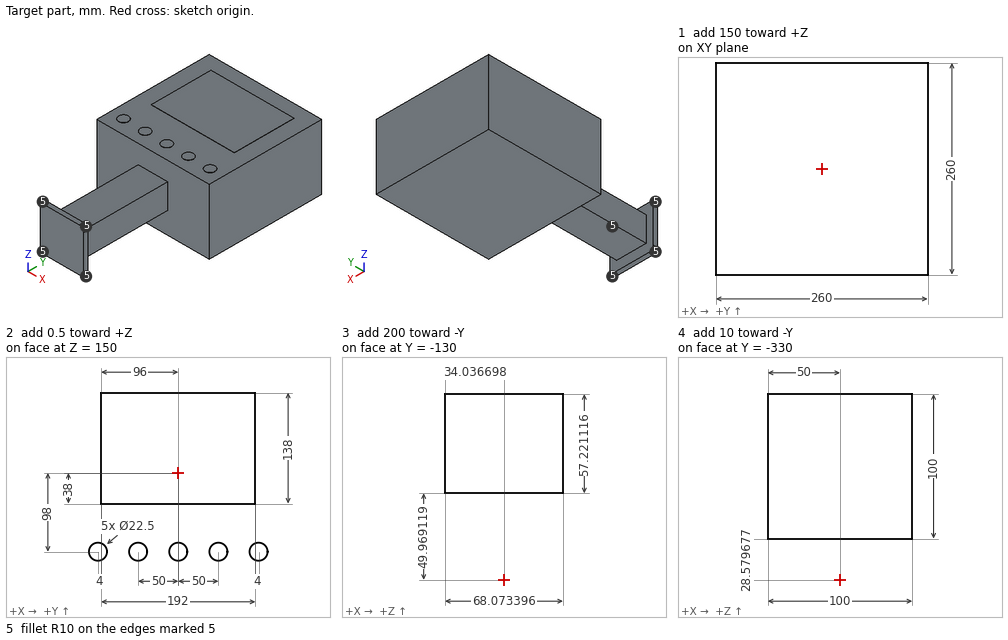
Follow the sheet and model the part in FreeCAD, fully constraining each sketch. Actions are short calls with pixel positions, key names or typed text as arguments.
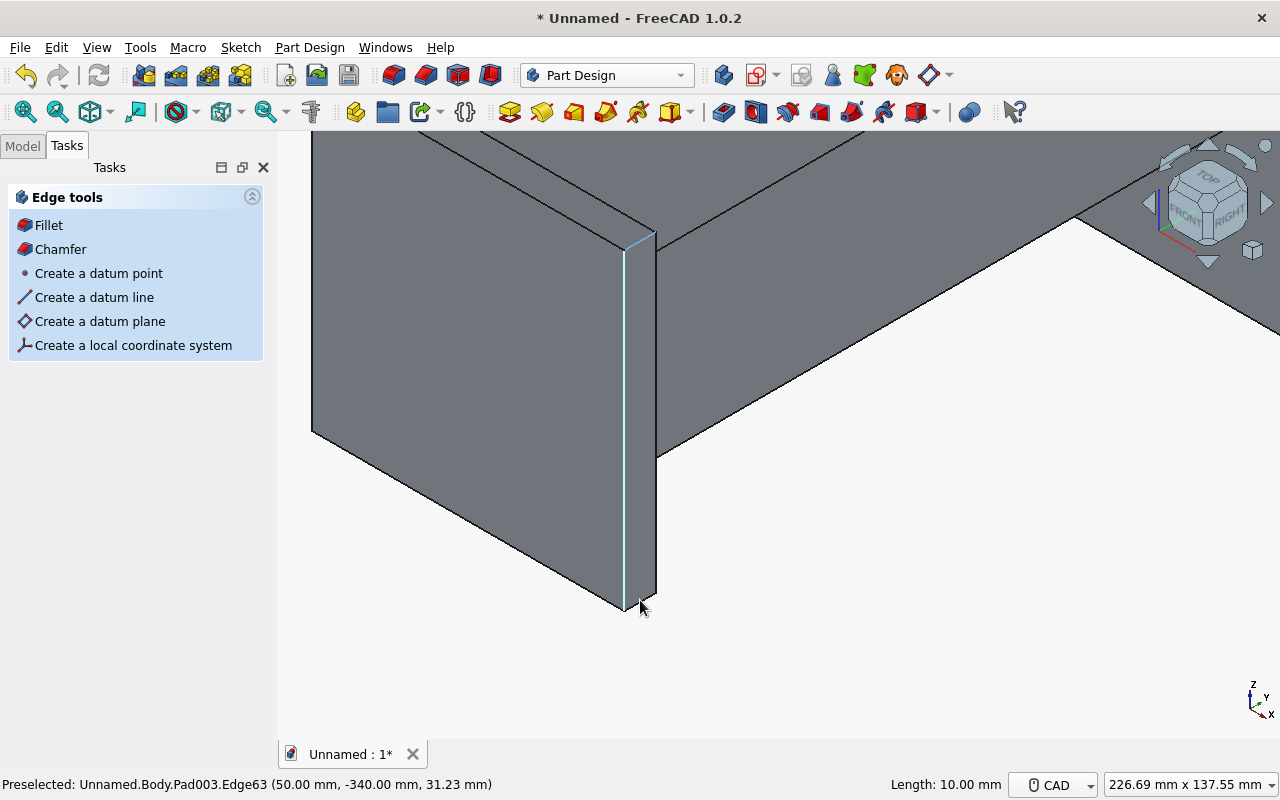
key(v)
key(f)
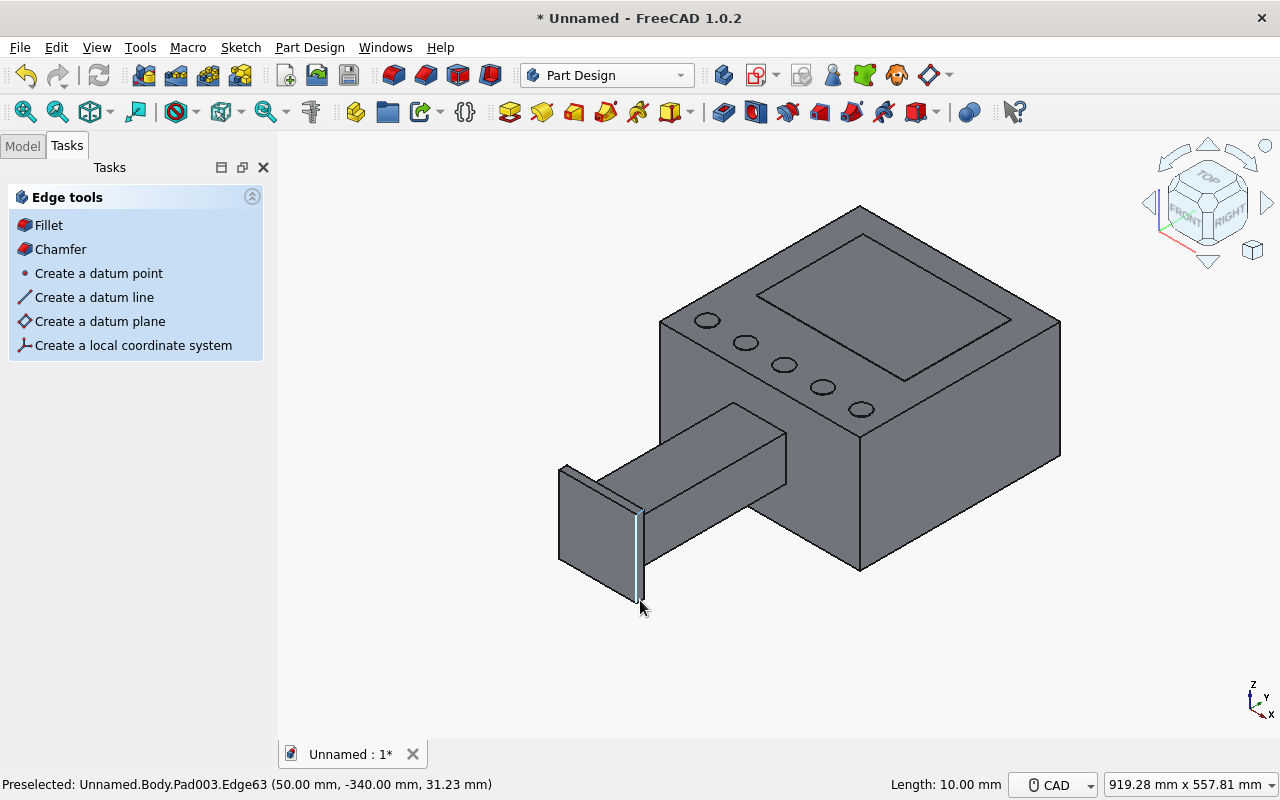
key(2)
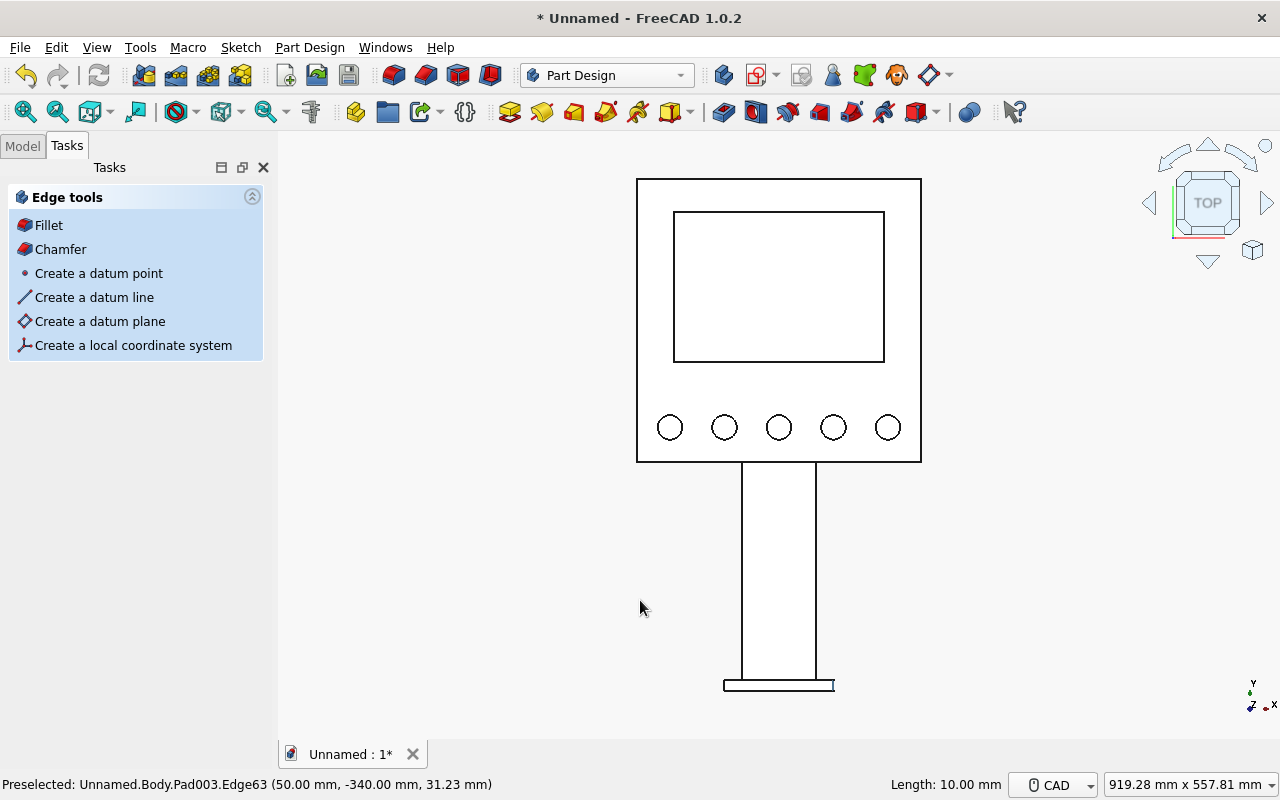
scroll(833, 685, up, 7)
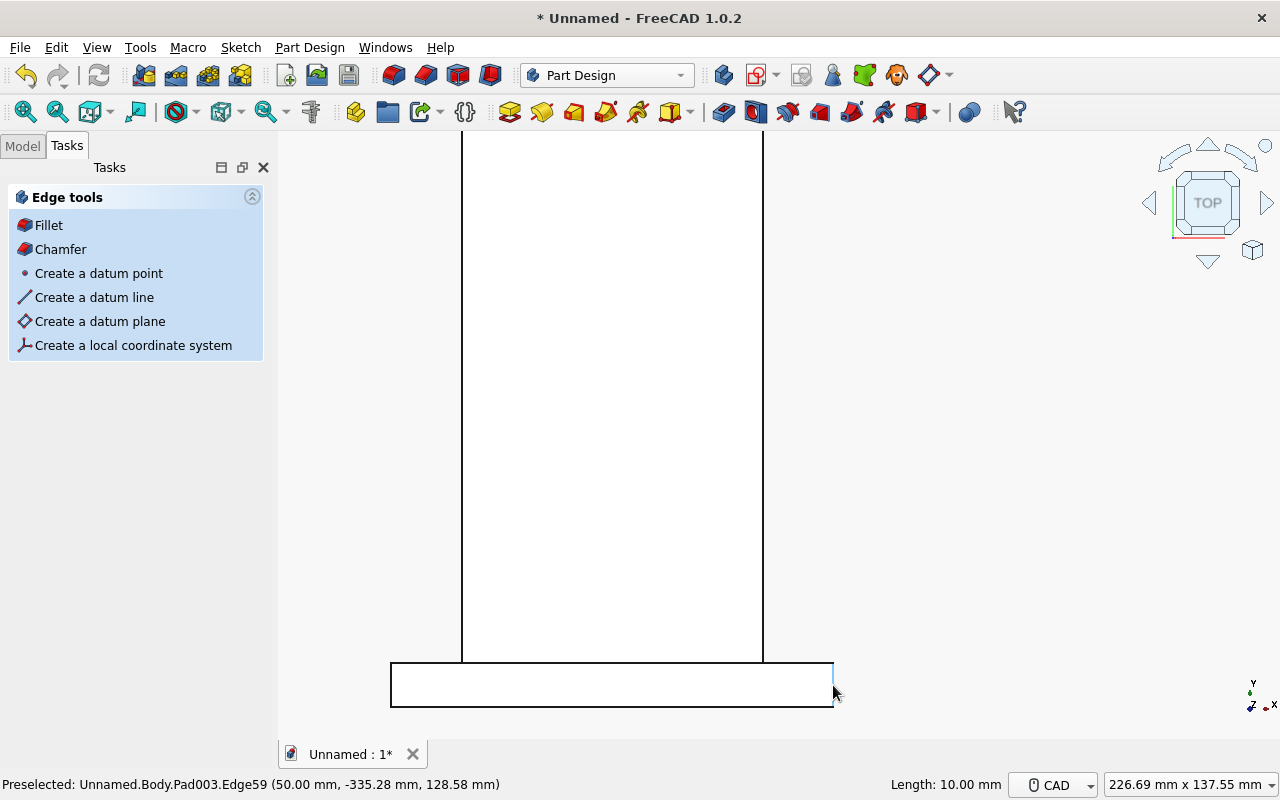
click(391, 684, ctrl)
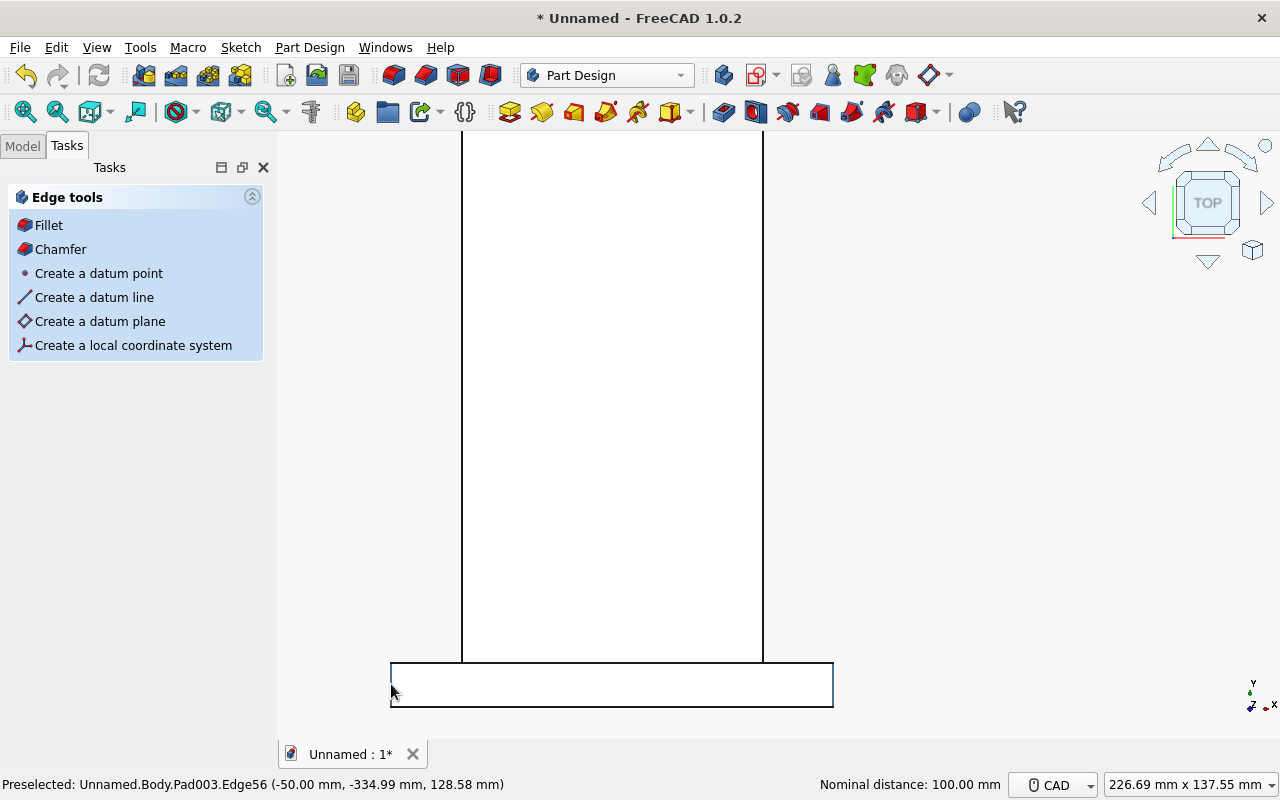
key(v)
key(f)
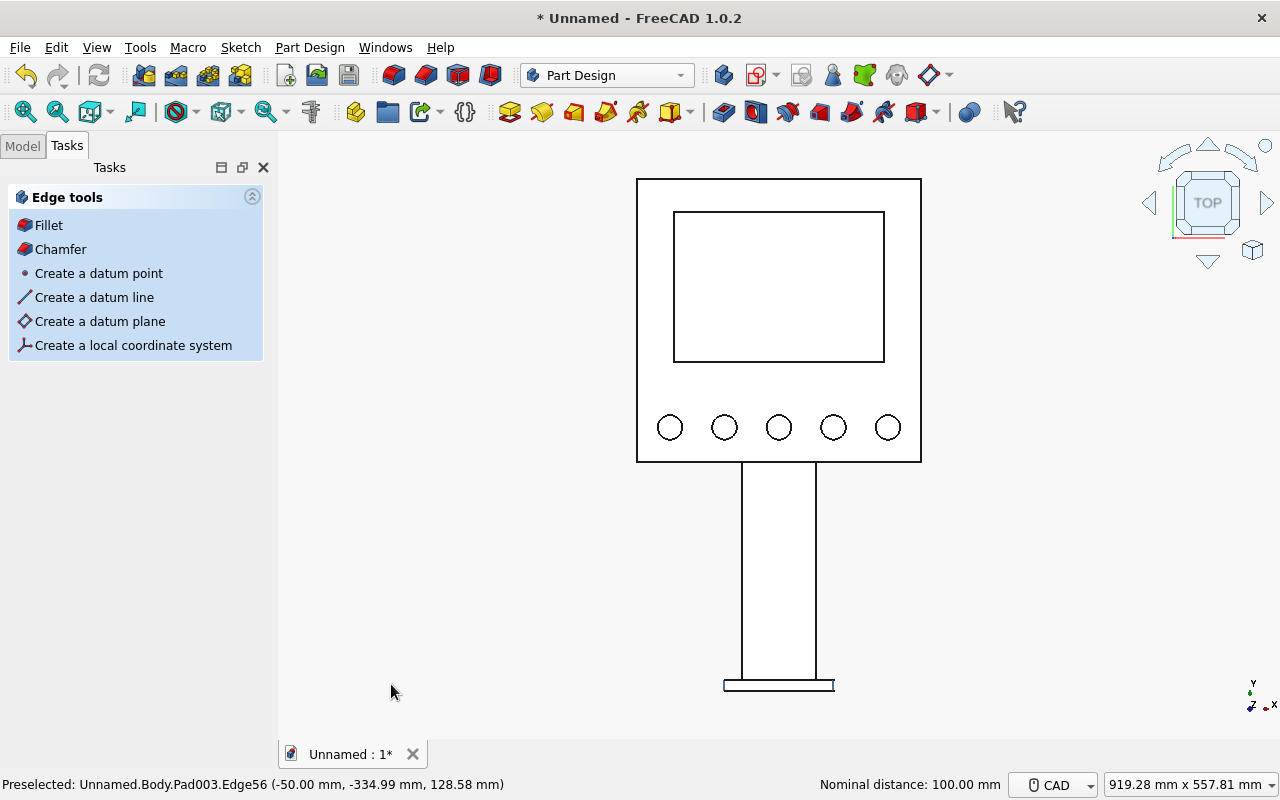
key(1)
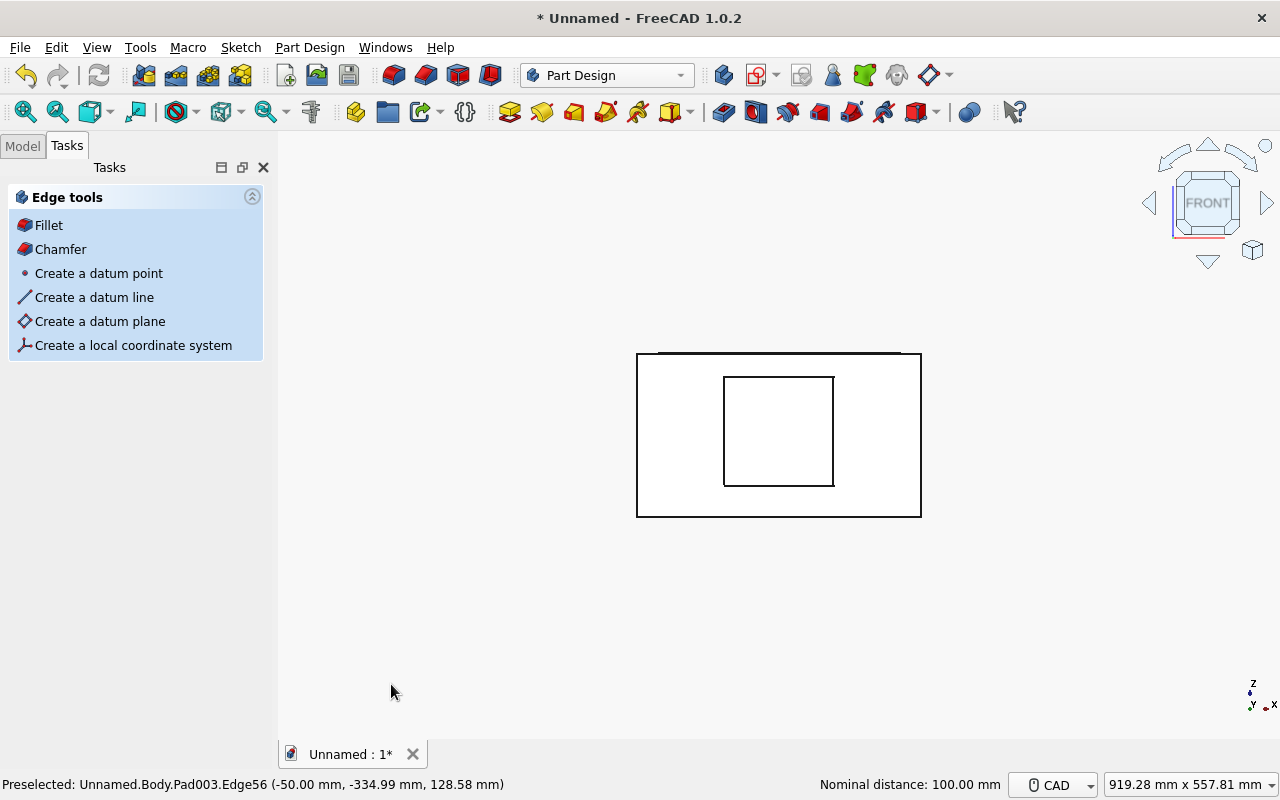
click(26, 112)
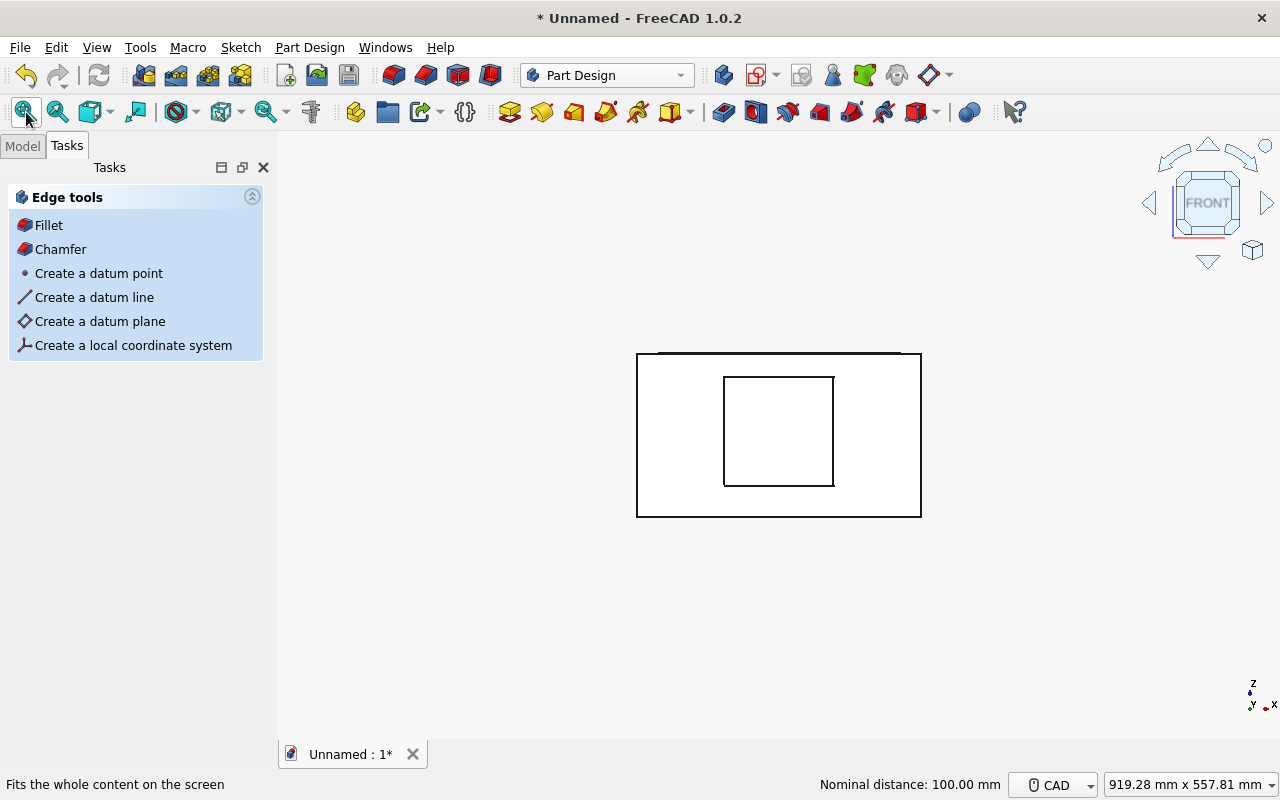
scroll(833, 485, up, 7)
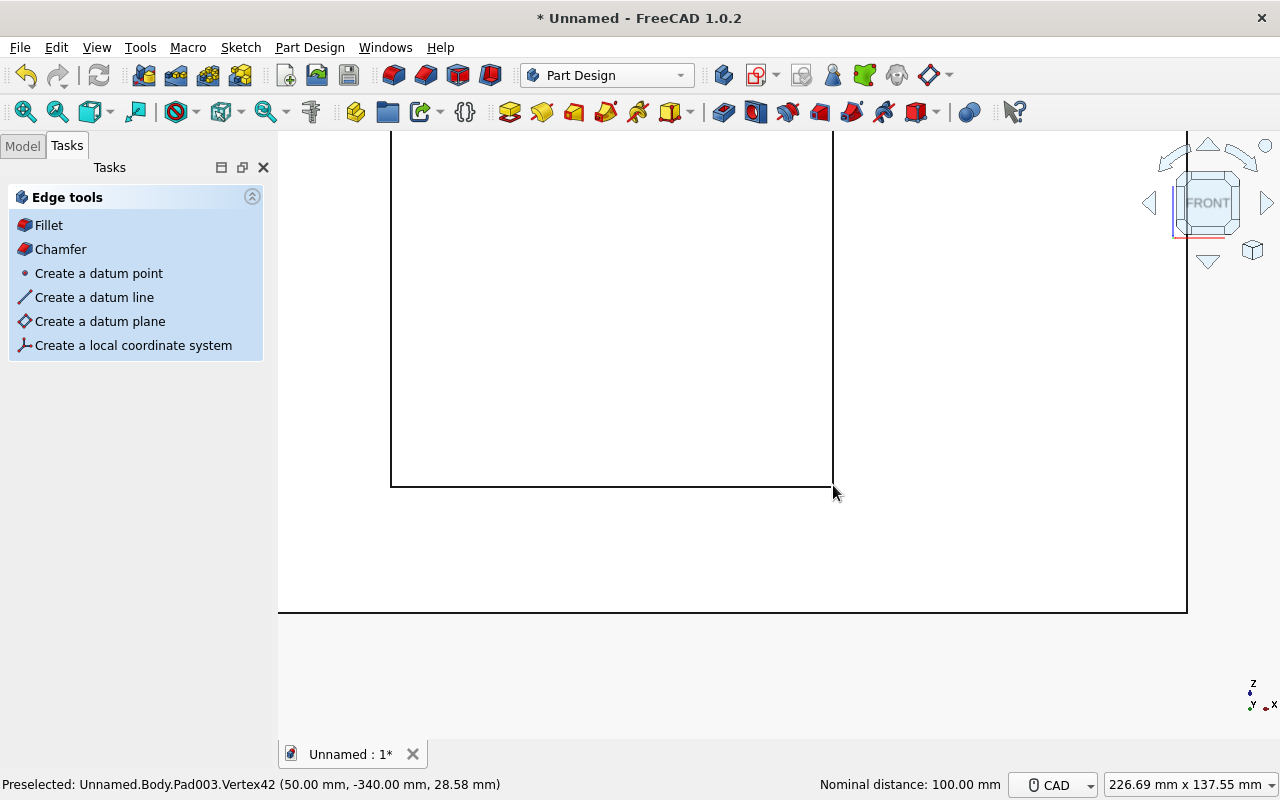
click(26, 112)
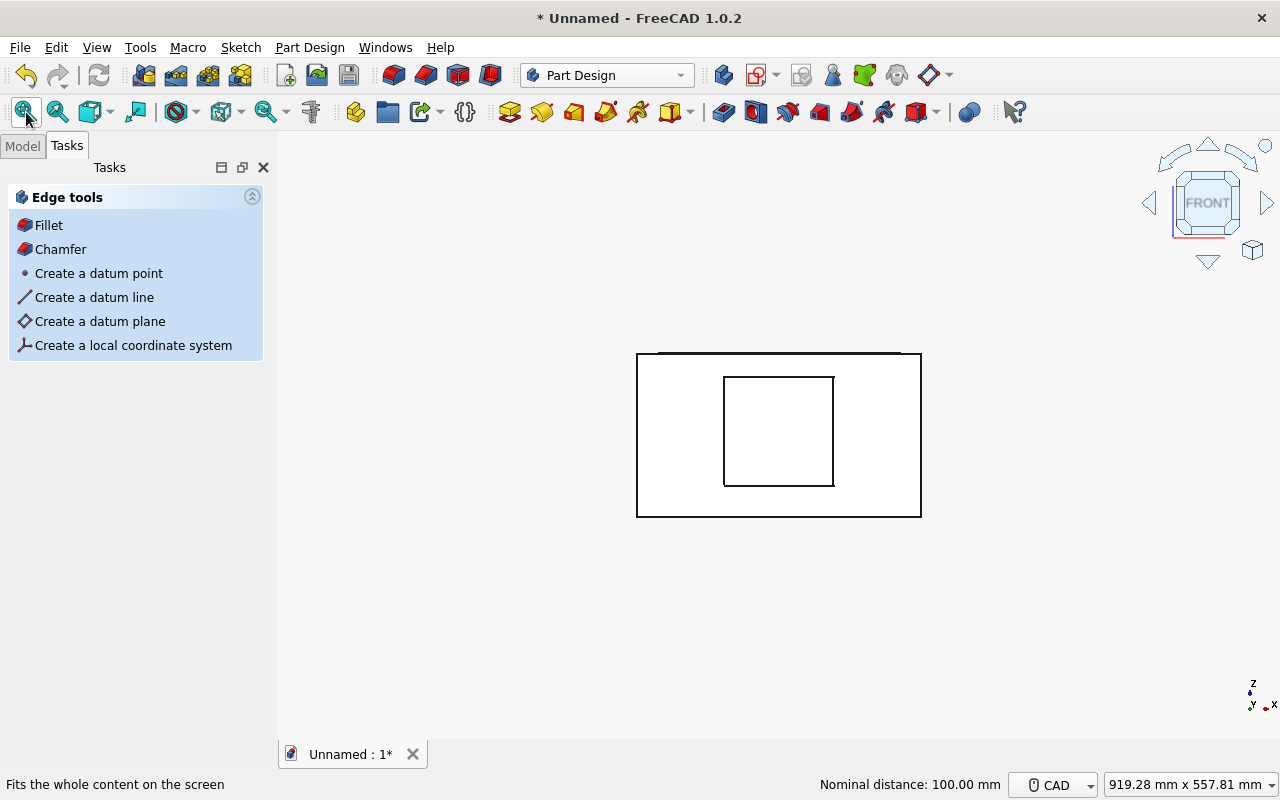
key(3)